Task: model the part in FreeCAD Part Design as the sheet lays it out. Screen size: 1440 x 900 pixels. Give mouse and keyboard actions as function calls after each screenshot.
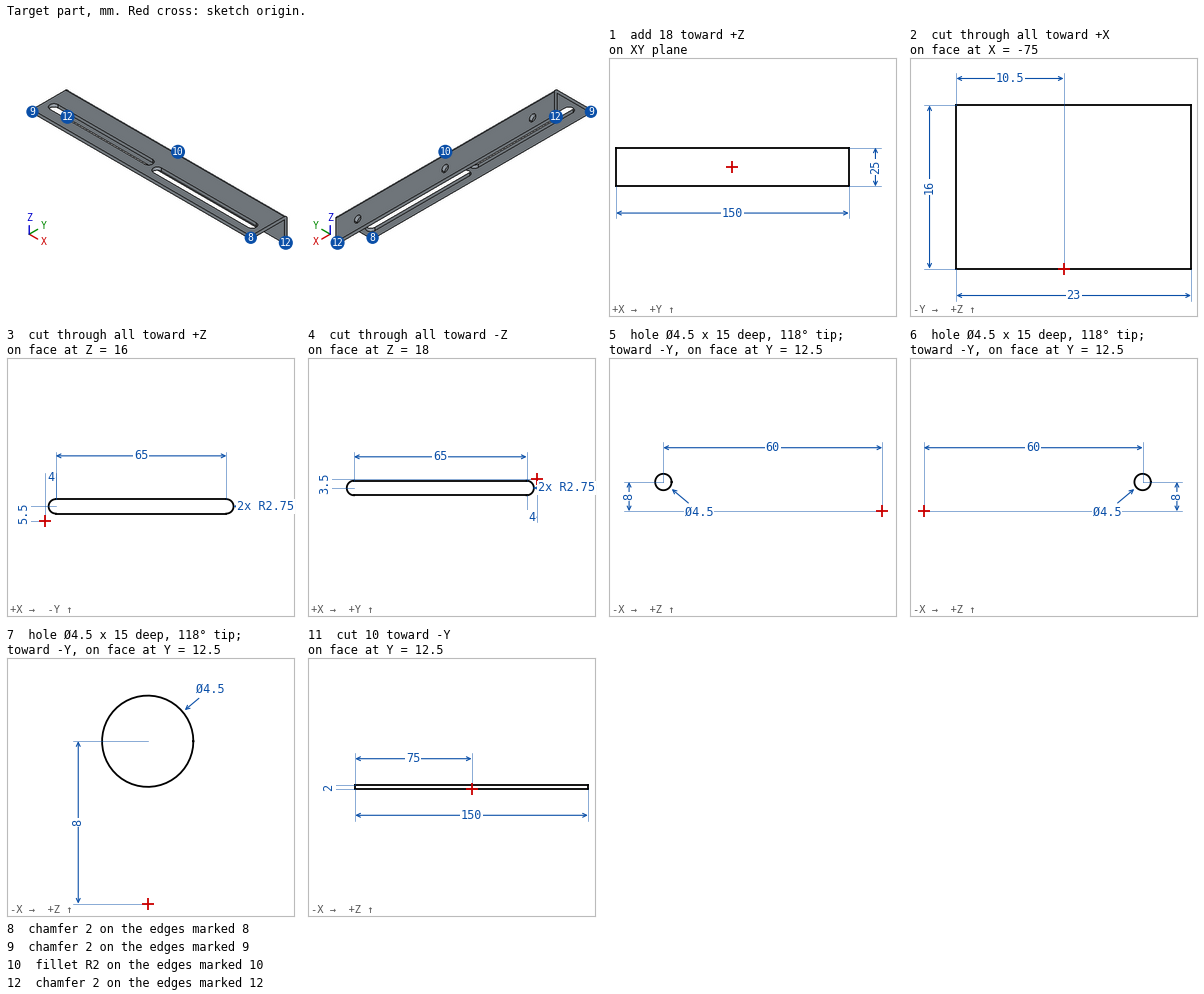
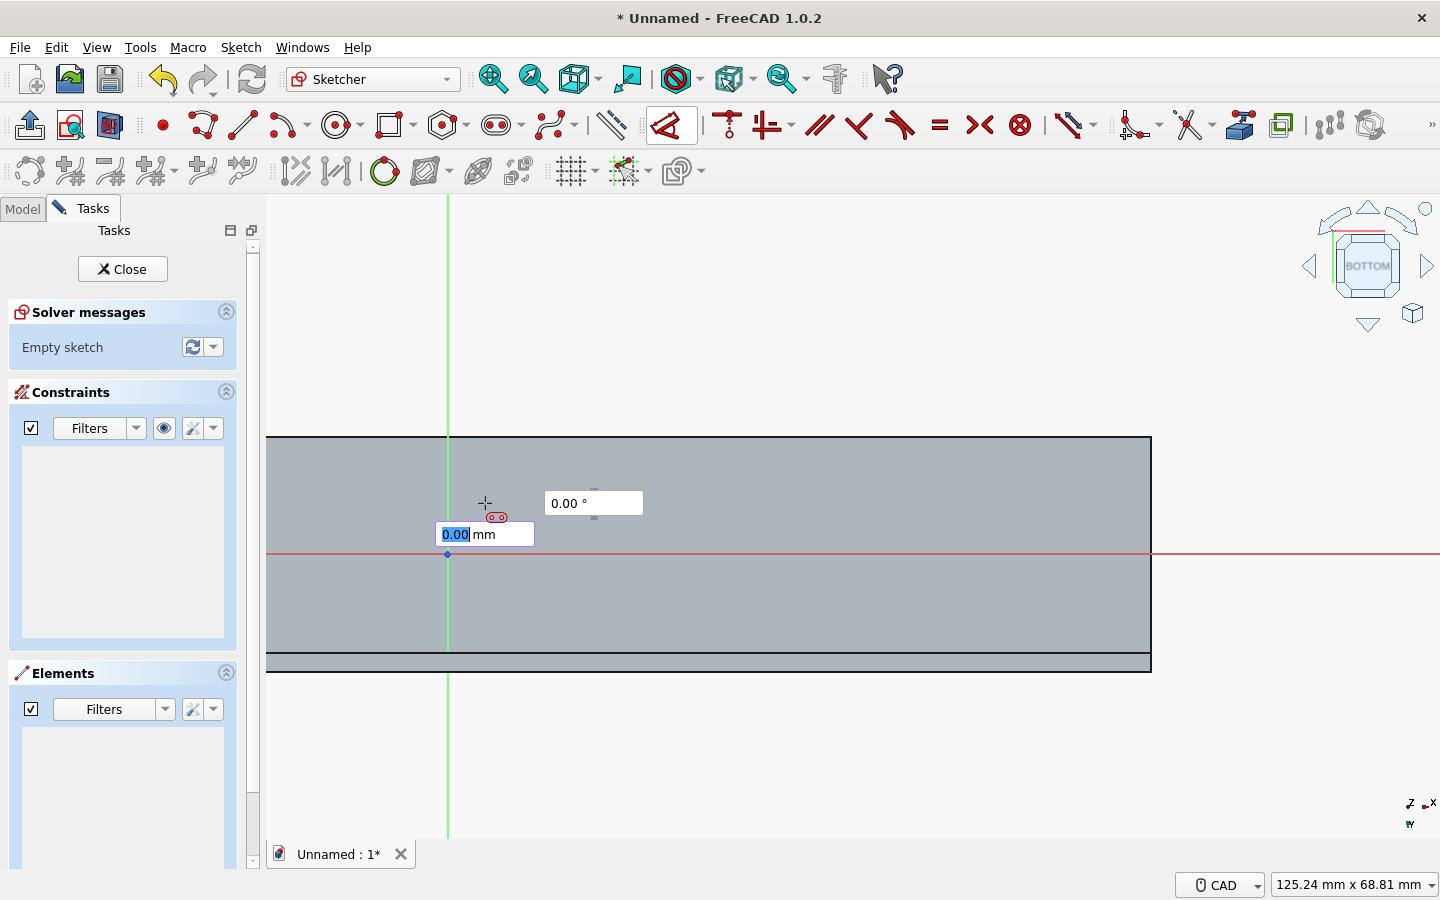
click(1094, 503)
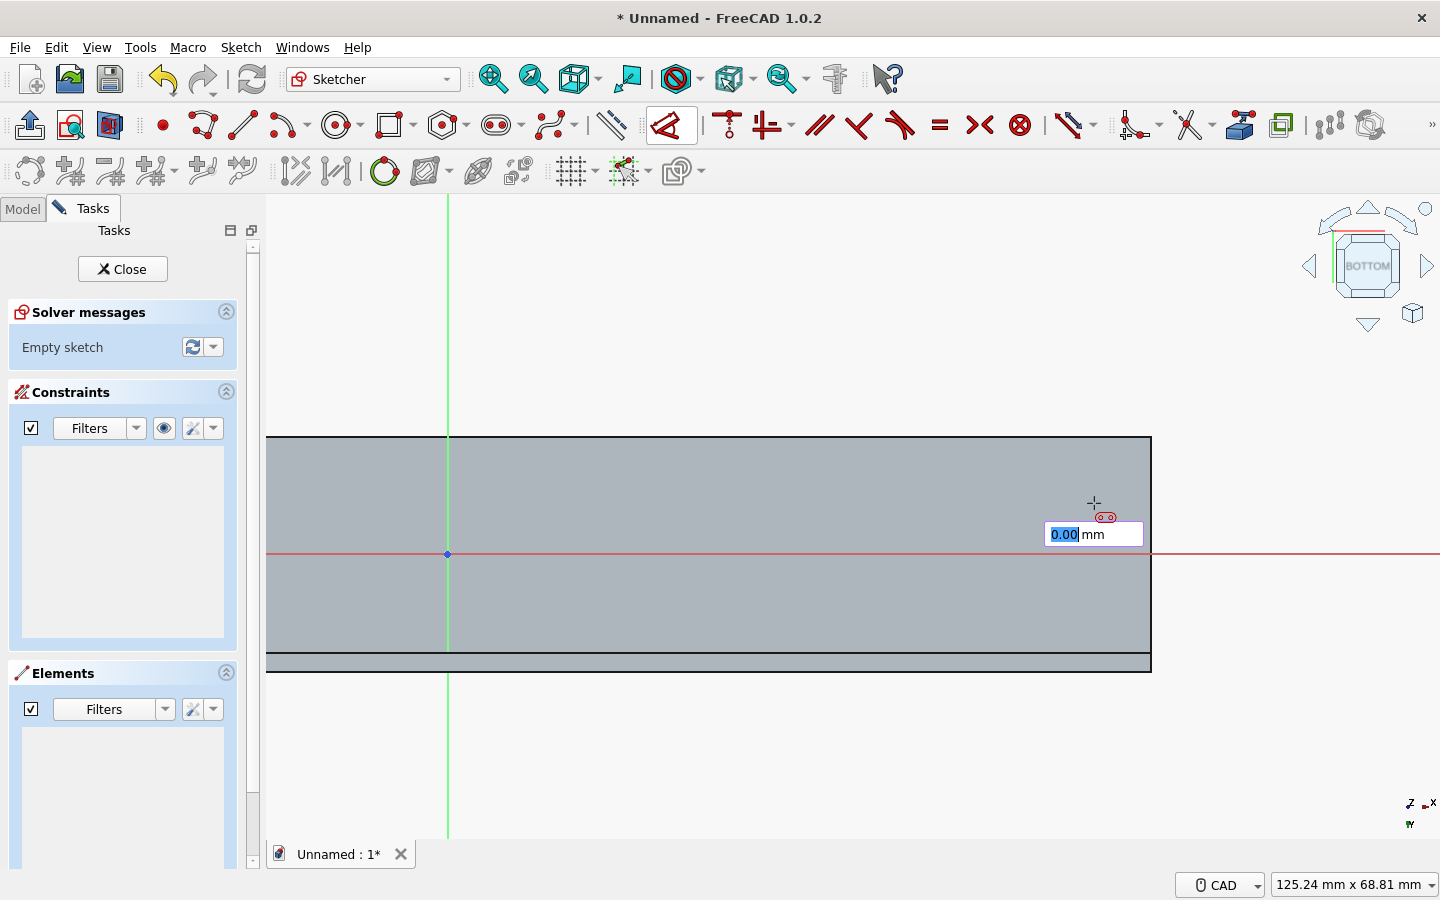
click(790, 529)
key(Escape)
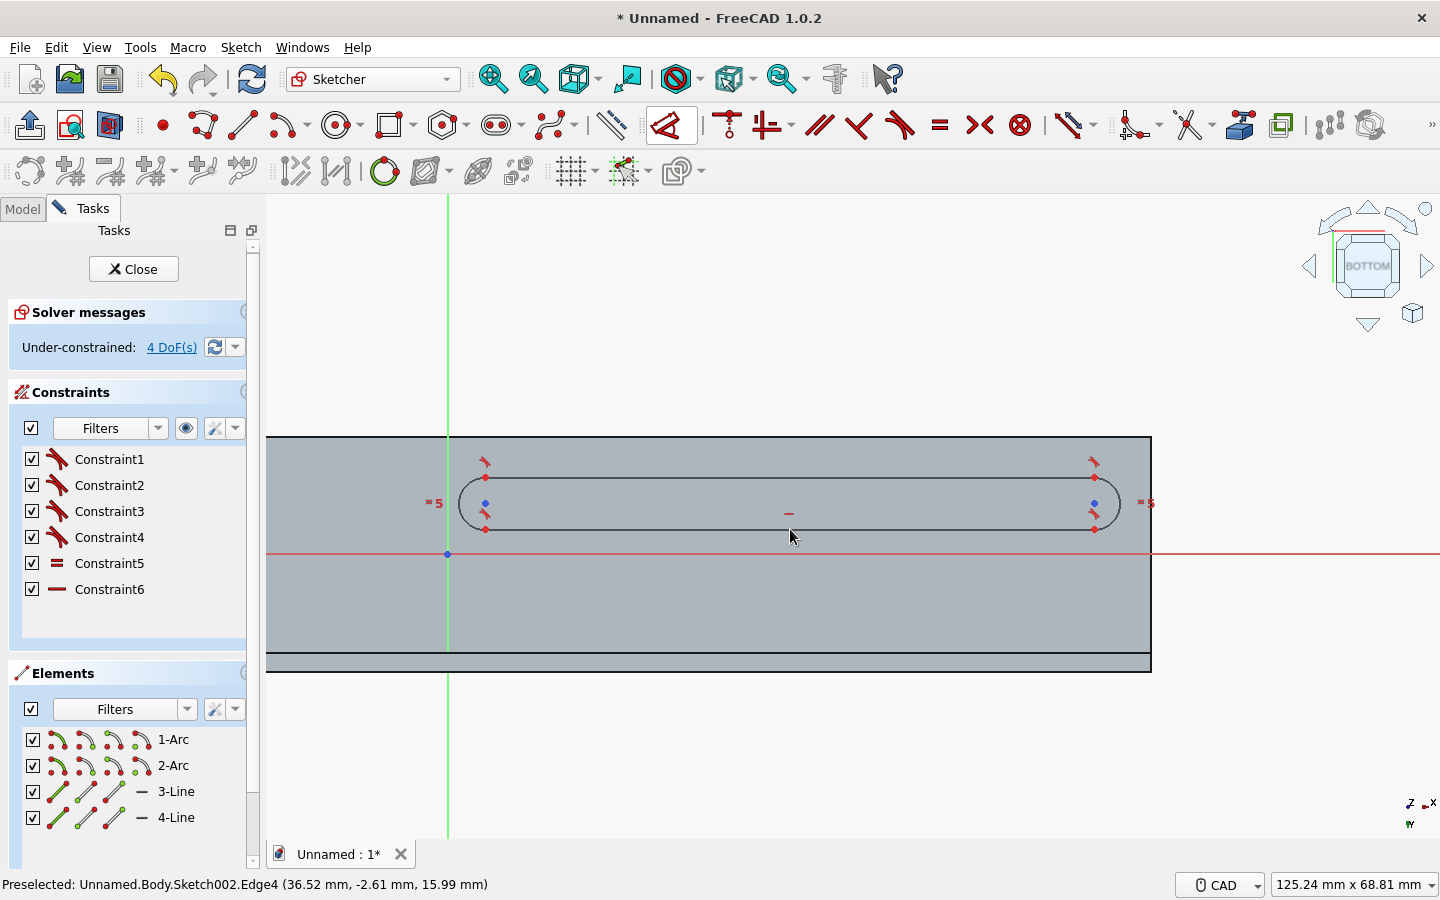
scroll(464, 489, up, 3)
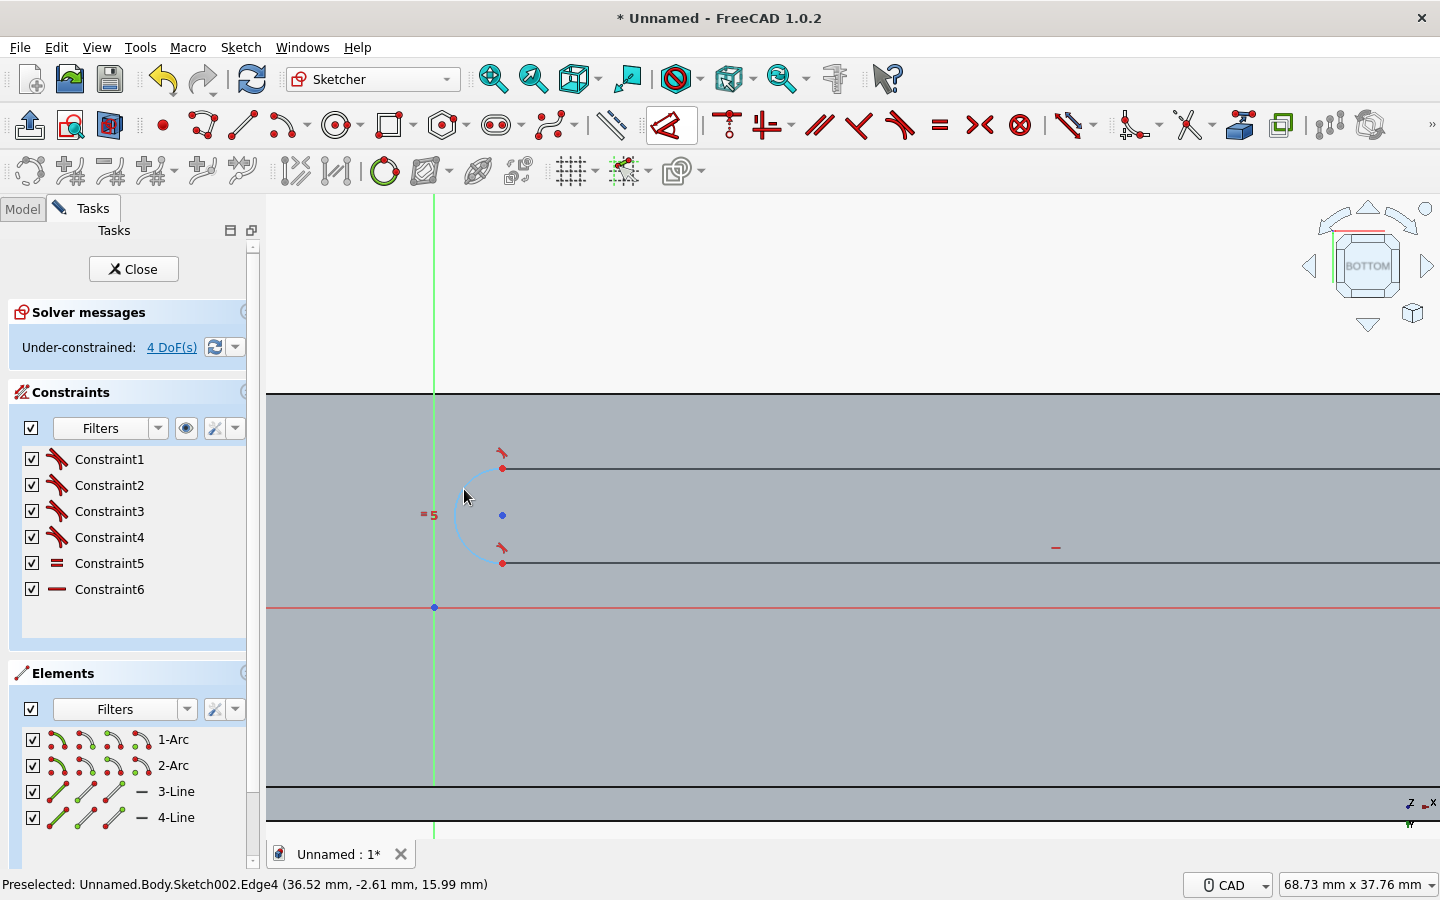
click(464, 488)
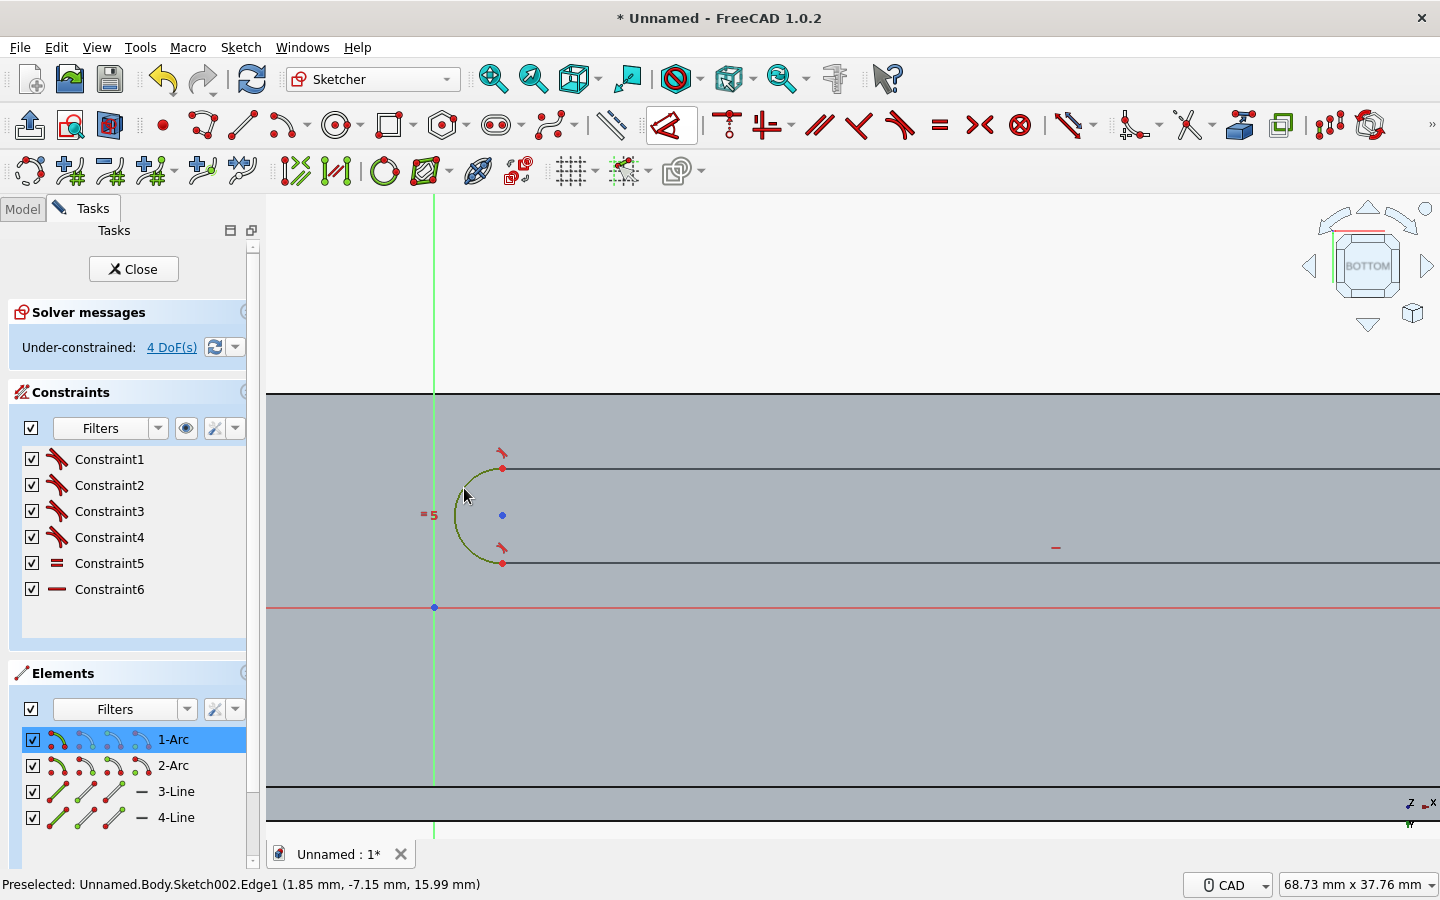
key(k)
key(r)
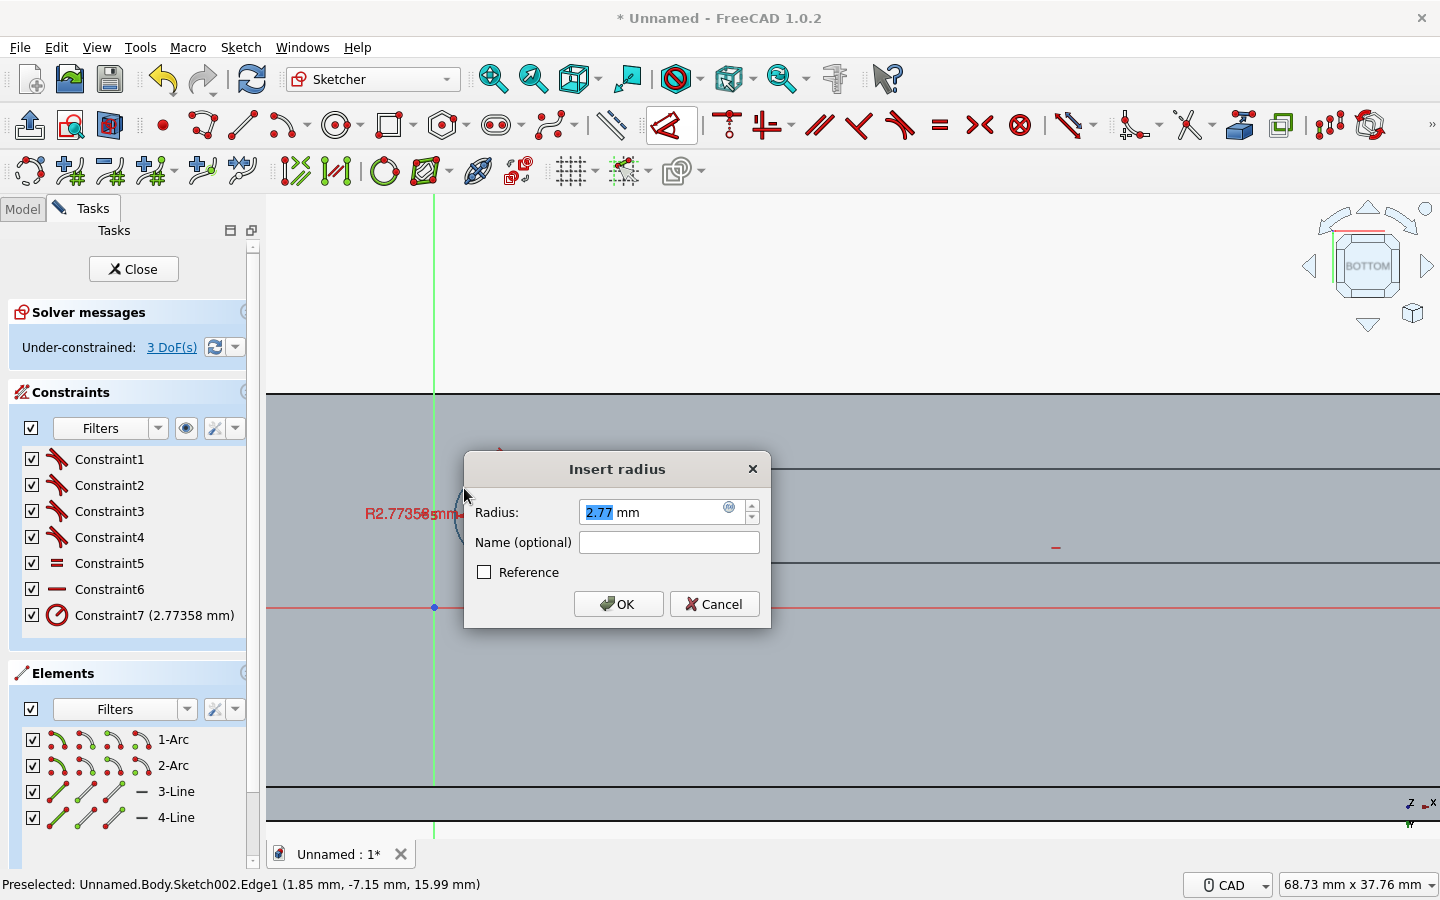
text(2.75)
key(Return)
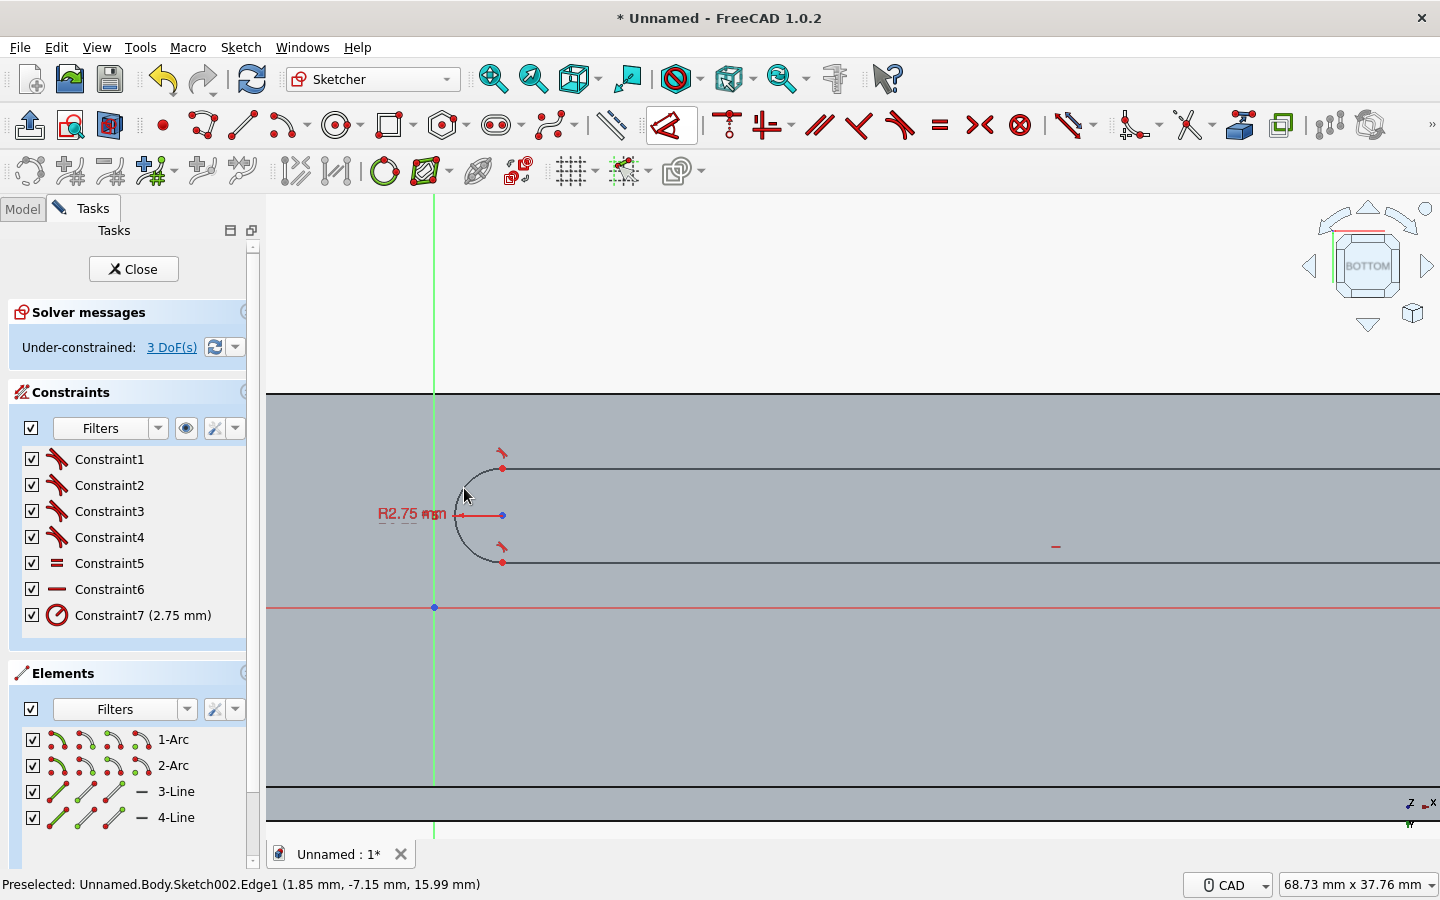
click(835, 469)